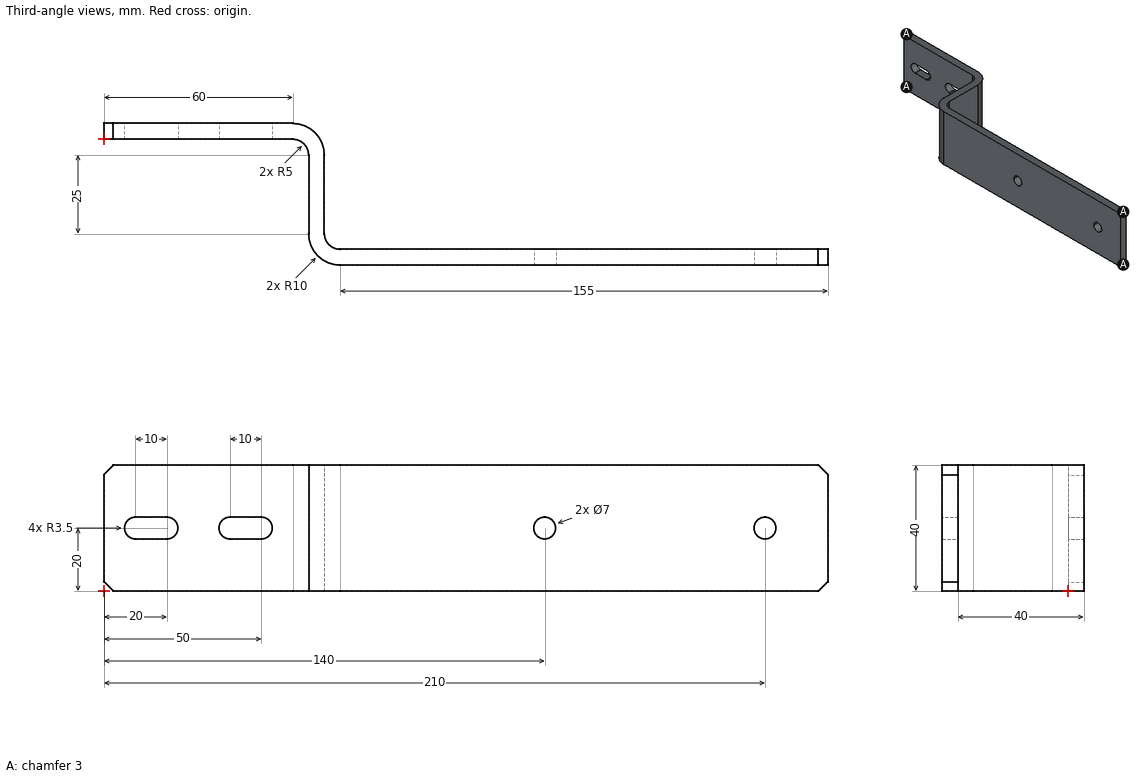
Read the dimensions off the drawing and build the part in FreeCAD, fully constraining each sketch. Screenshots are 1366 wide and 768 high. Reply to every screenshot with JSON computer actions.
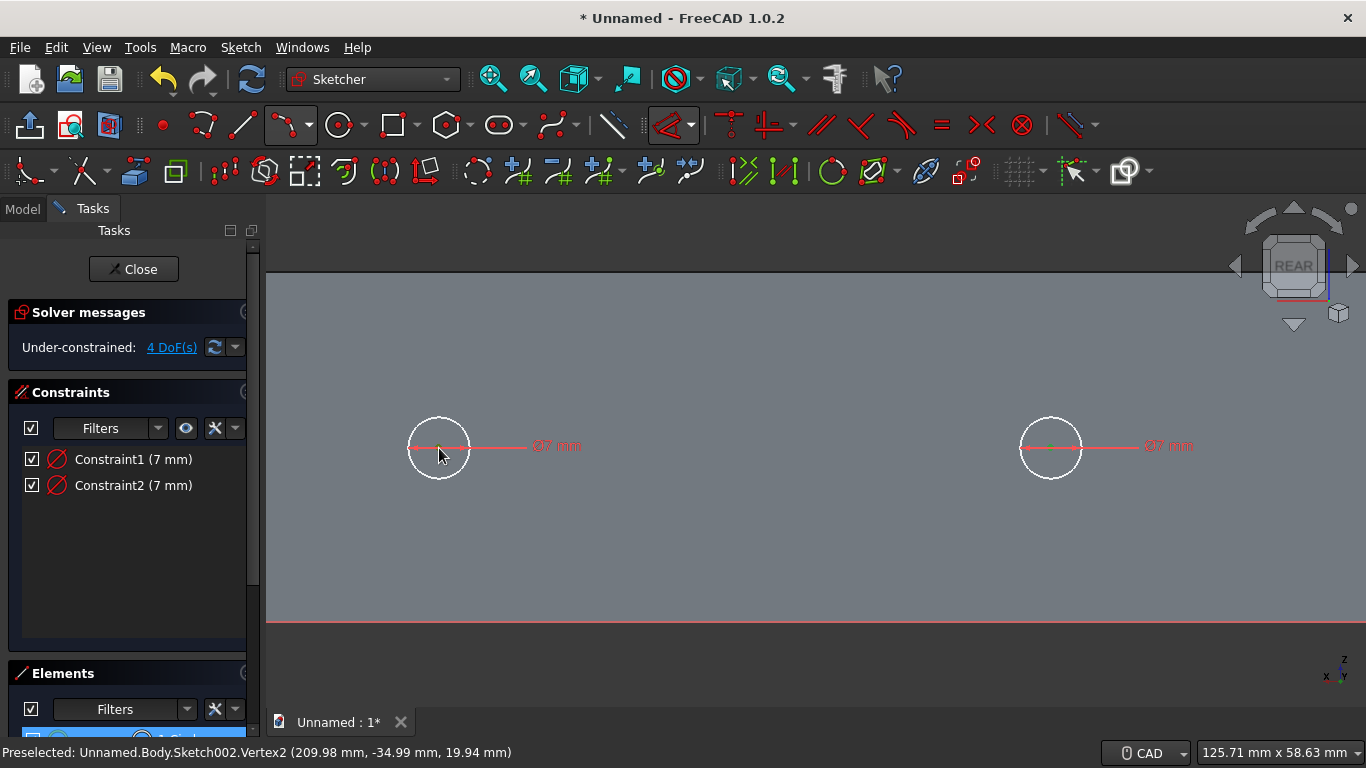
{"action": "left_click", "coordinate": [796, 126]}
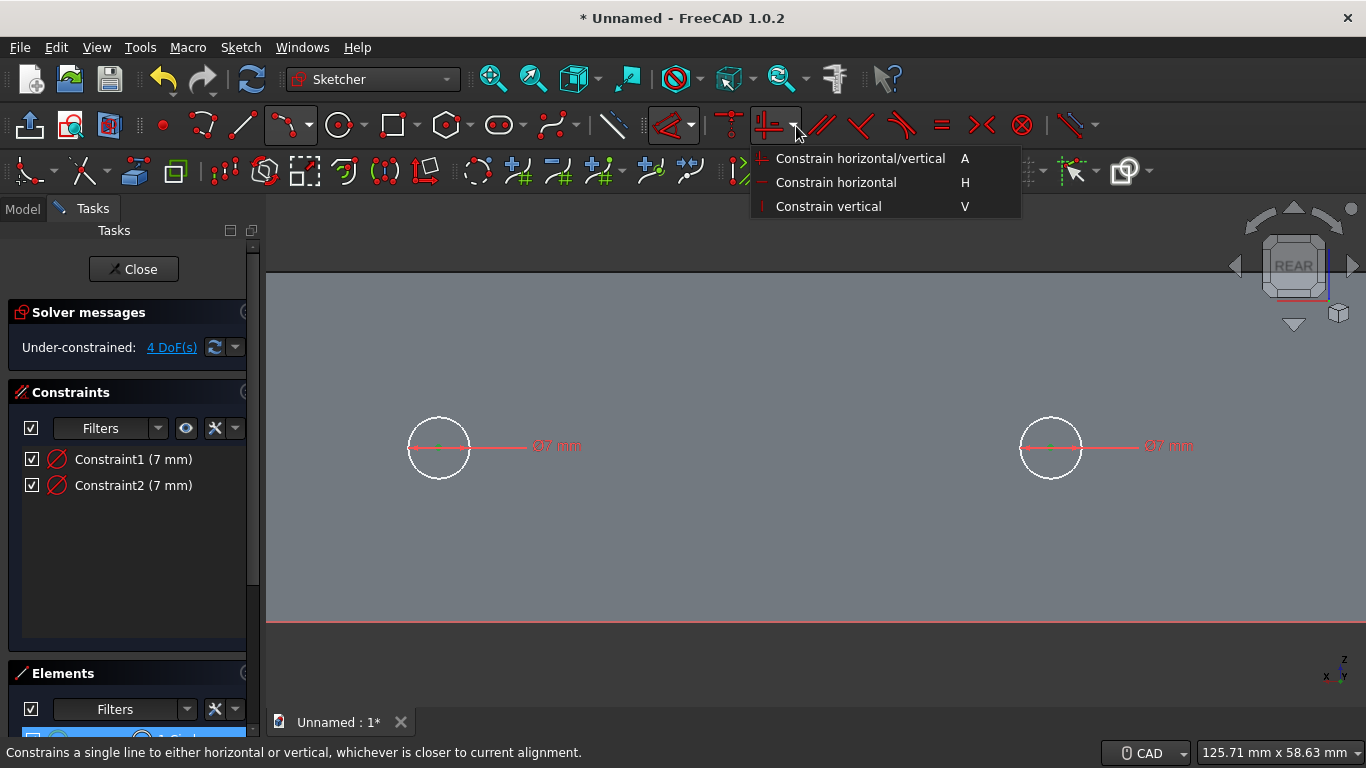
{"action": "left_click", "coordinate": [886, 182]}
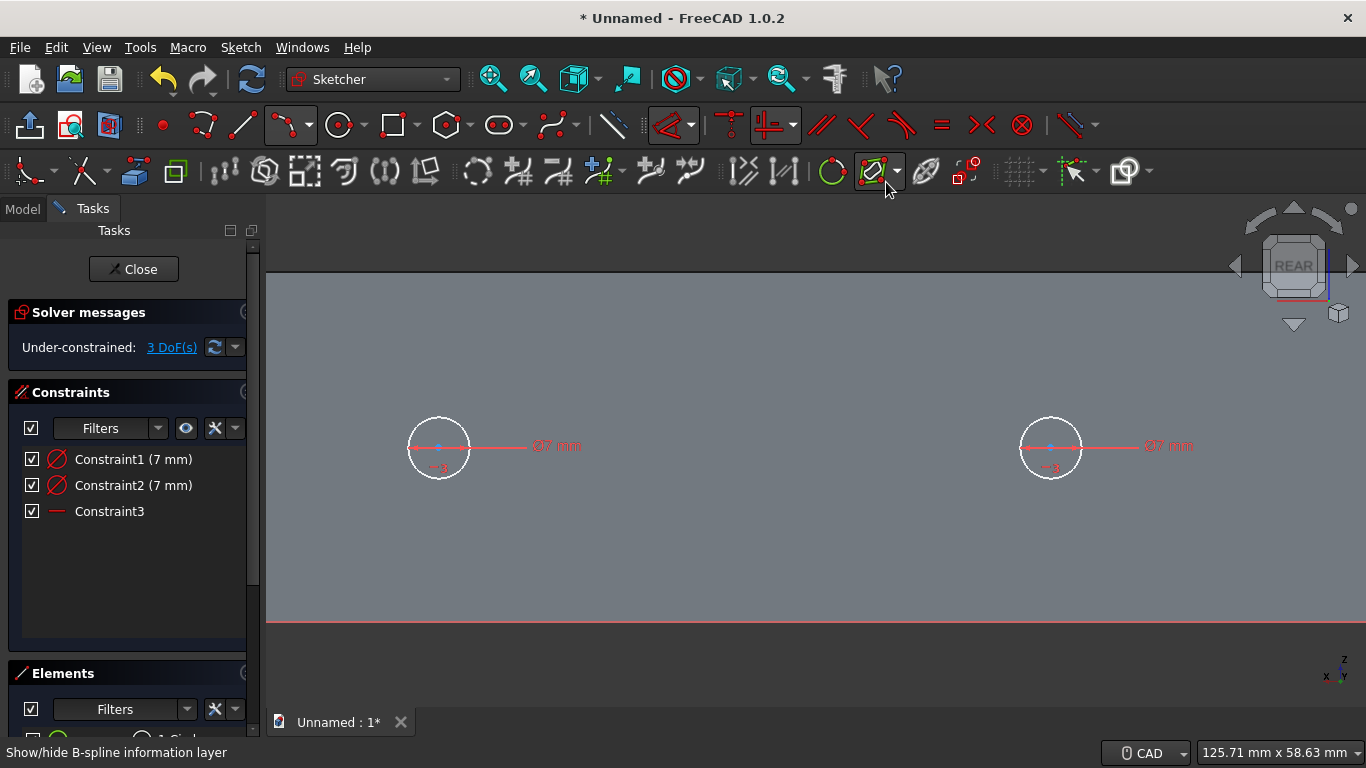
{"action": "left_click", "coordinate": [1051, 448]}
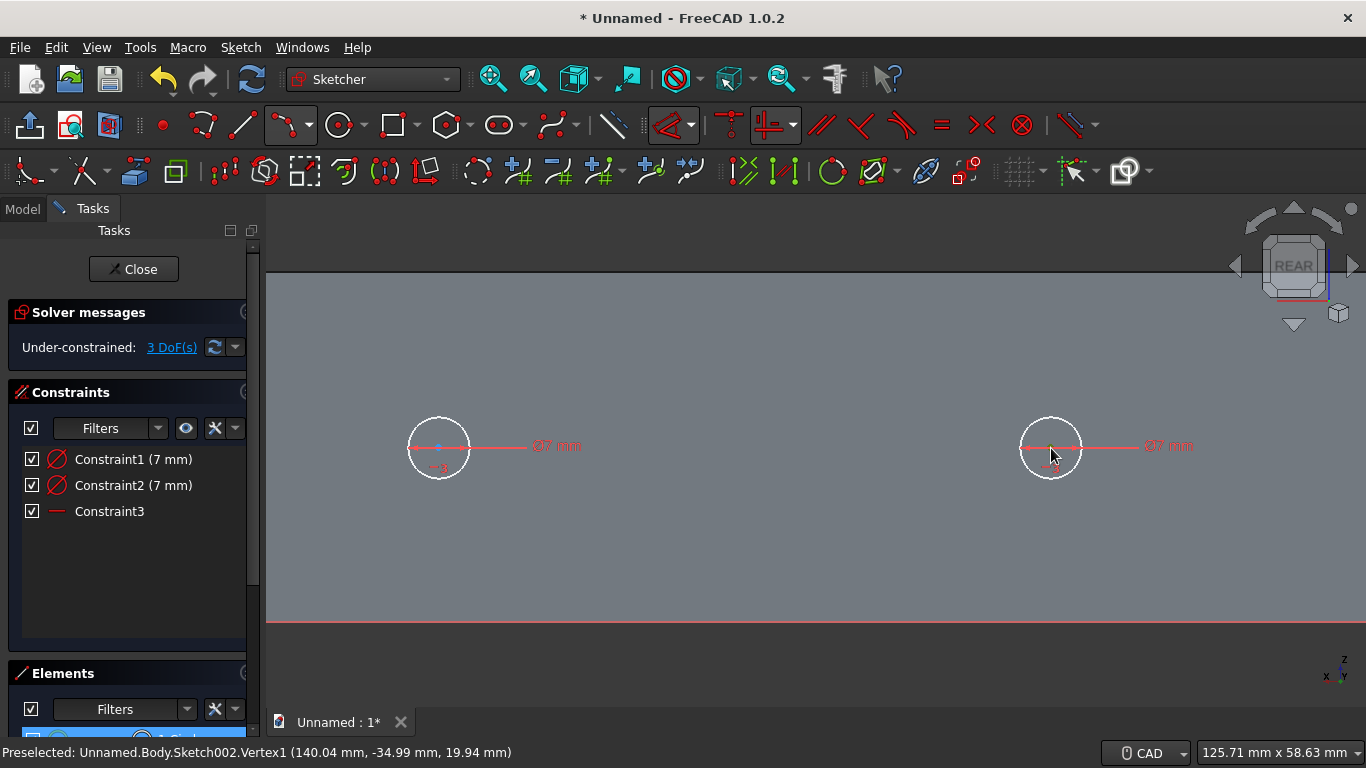
{"action": "key", "text": "i"}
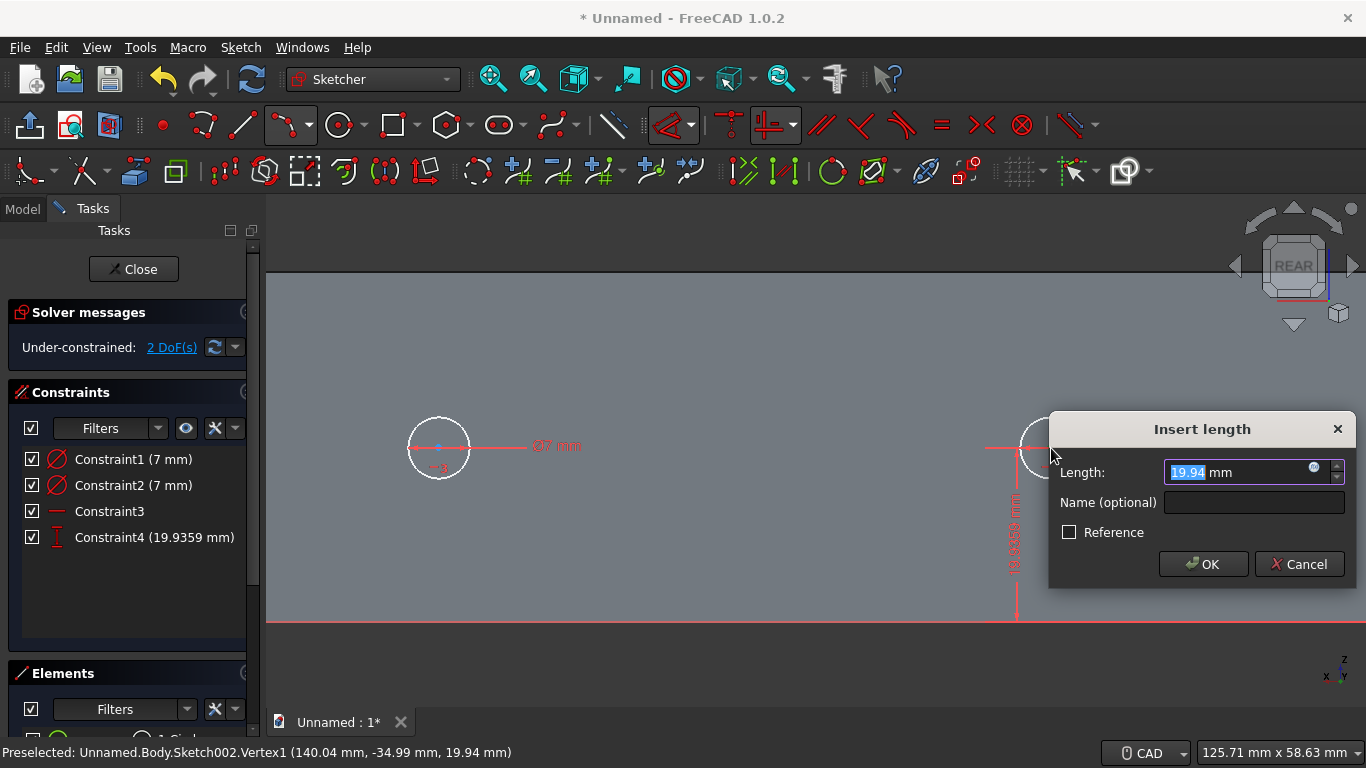
{"action": "type", "text": "20"}
{"action": "key", "text": "Return"}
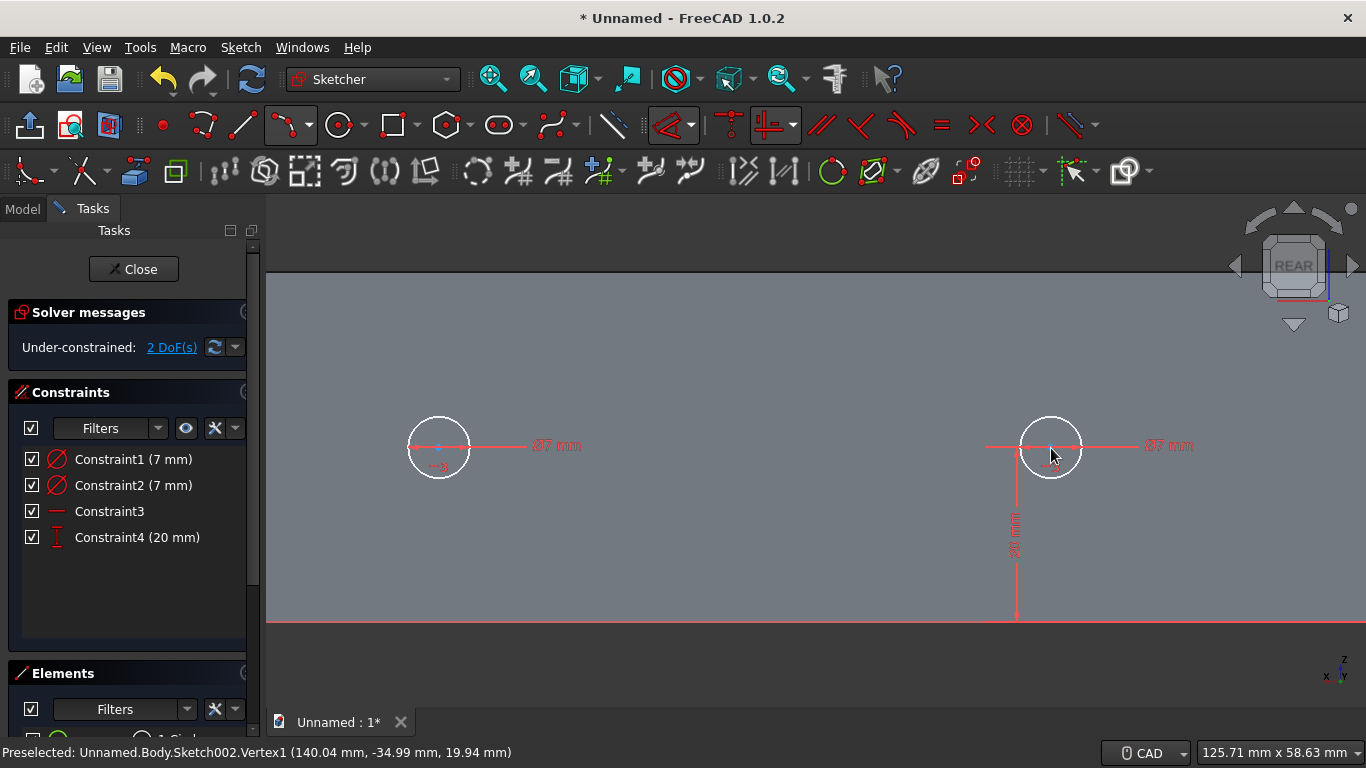
{"action": "left_click", "coordinate": [1051, 447]}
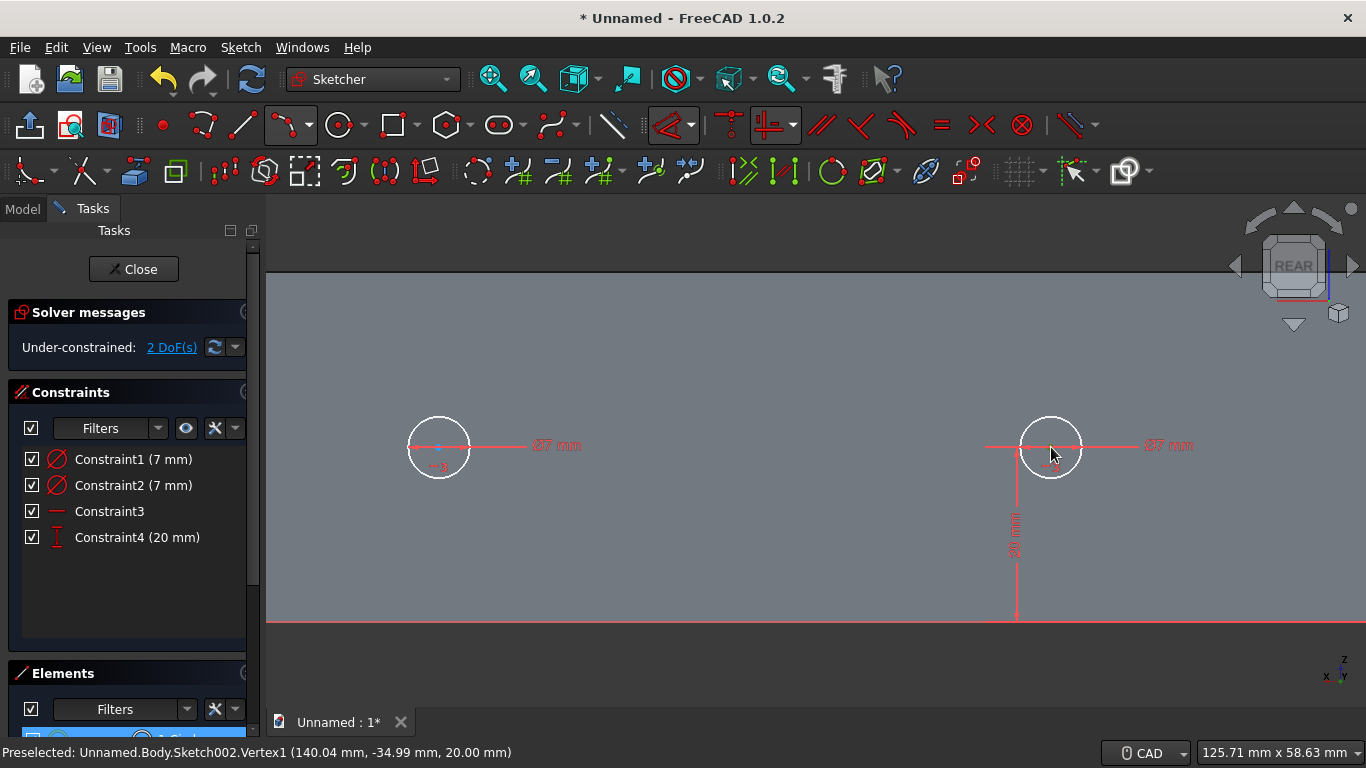
{"action": "key", "text": "l"}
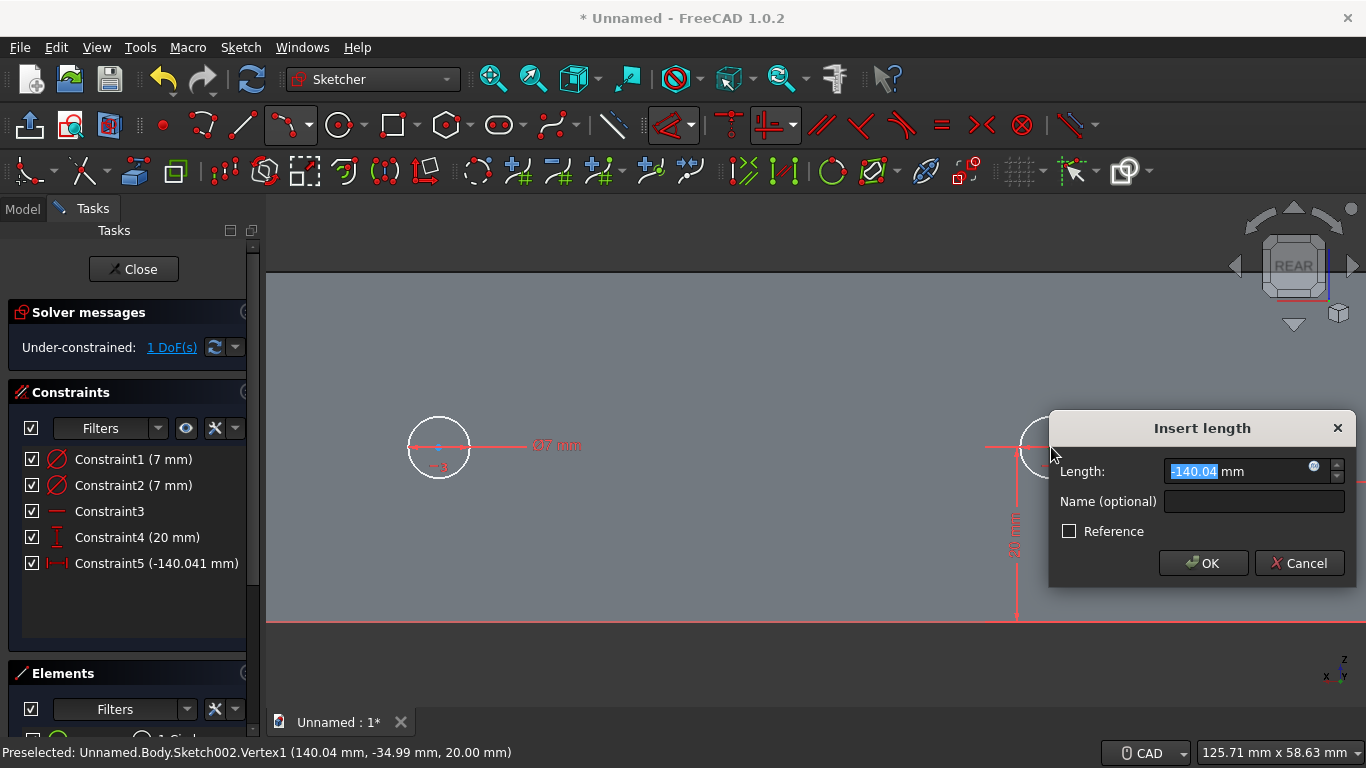
{"action": "type", "text": "-140"}
{"action": "key", "text": "Return"}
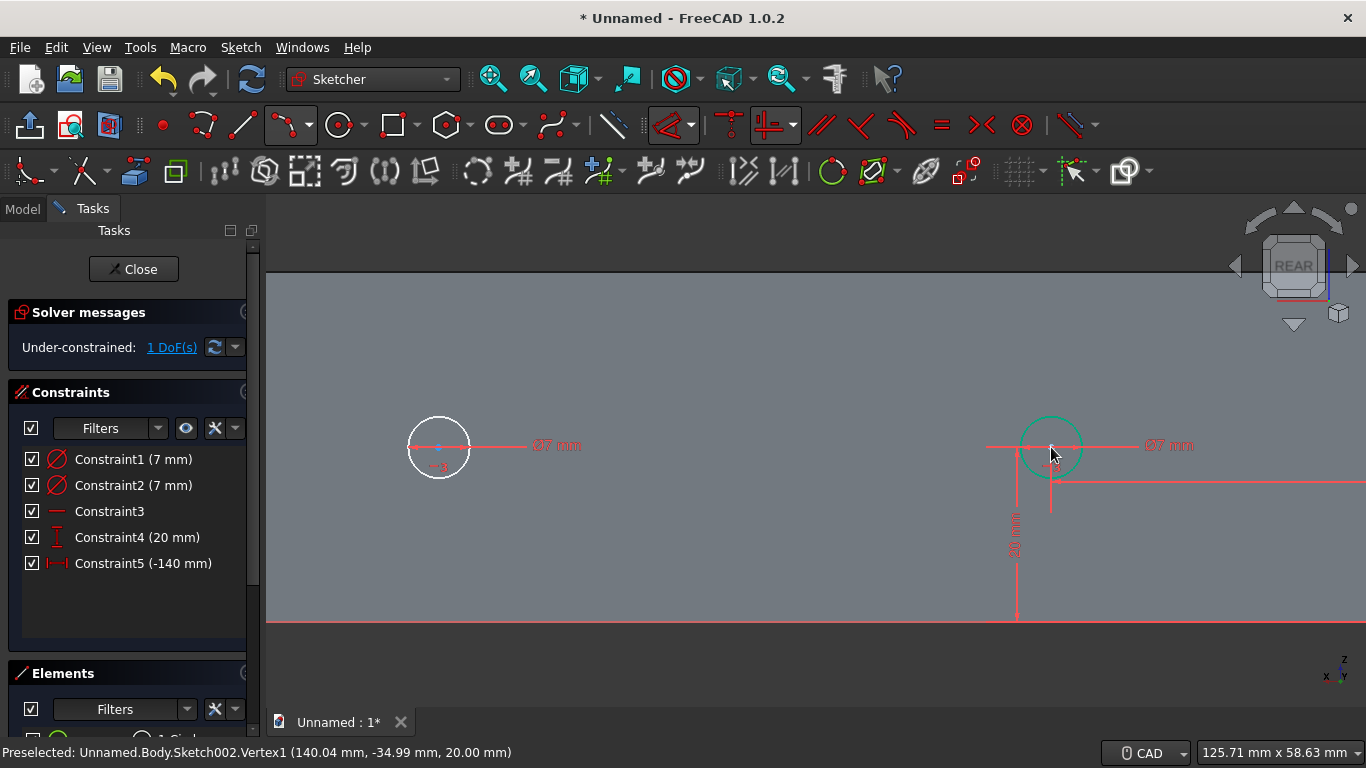
{"action": "left_click", "coordinate": [439, 447]}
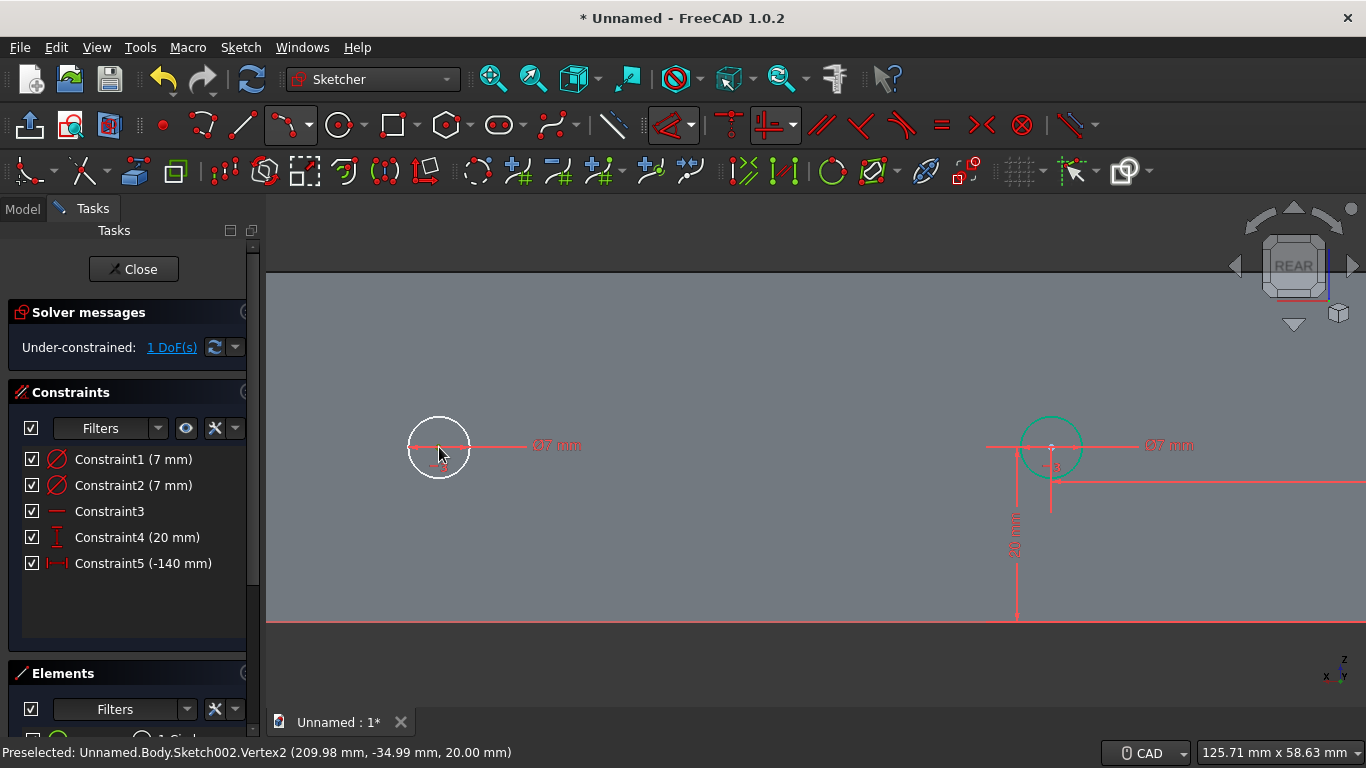
{"action": "key", "text": "l"}